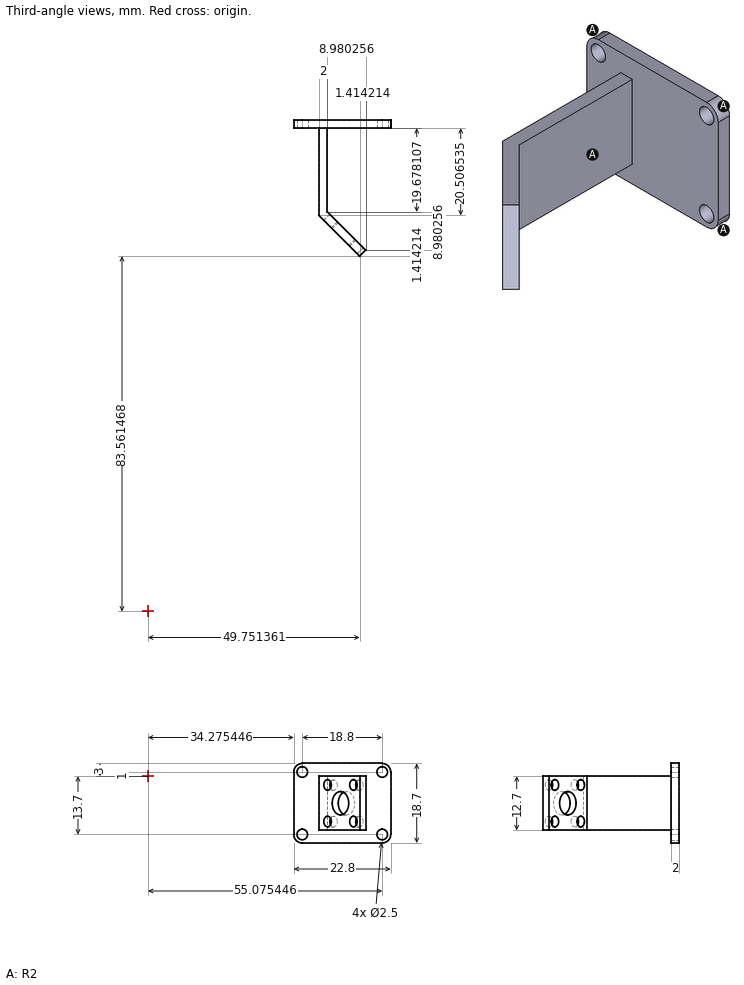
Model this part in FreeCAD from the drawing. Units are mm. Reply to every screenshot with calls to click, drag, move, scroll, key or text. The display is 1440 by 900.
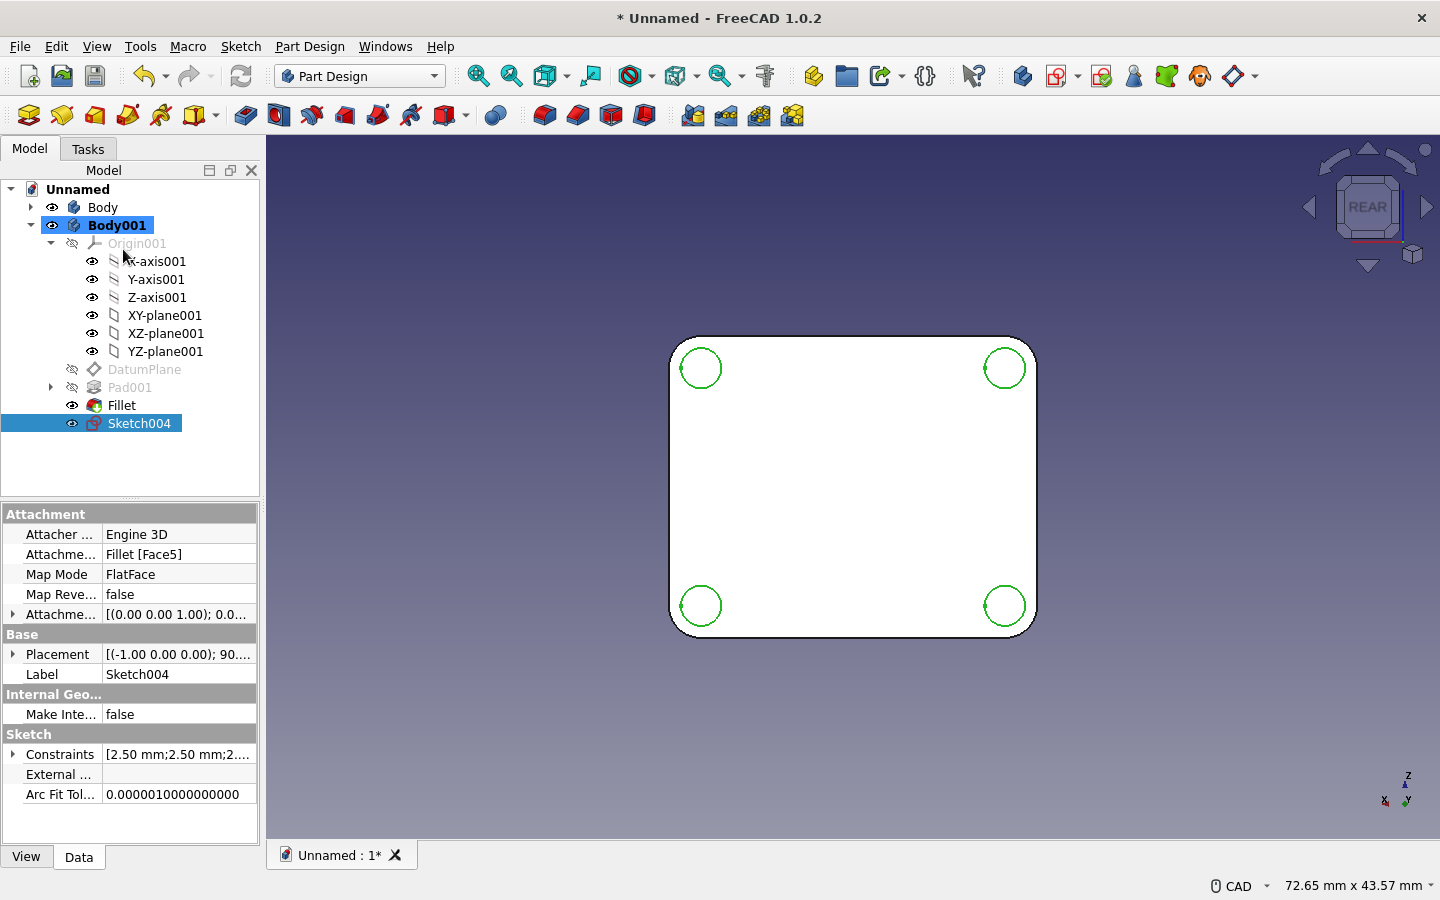
click(246, 116)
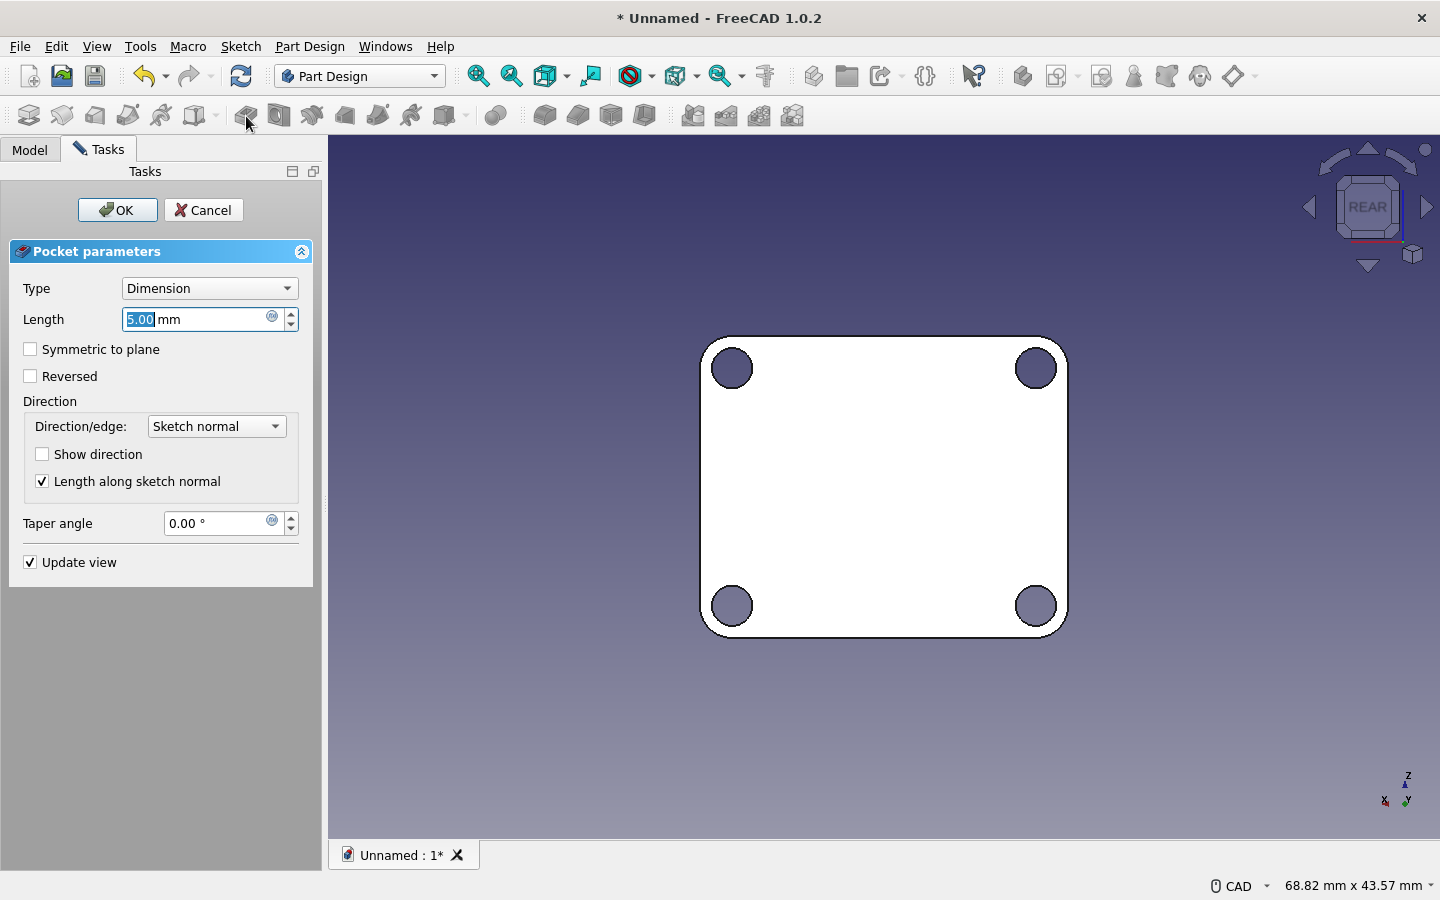
text(2)
key(Tab)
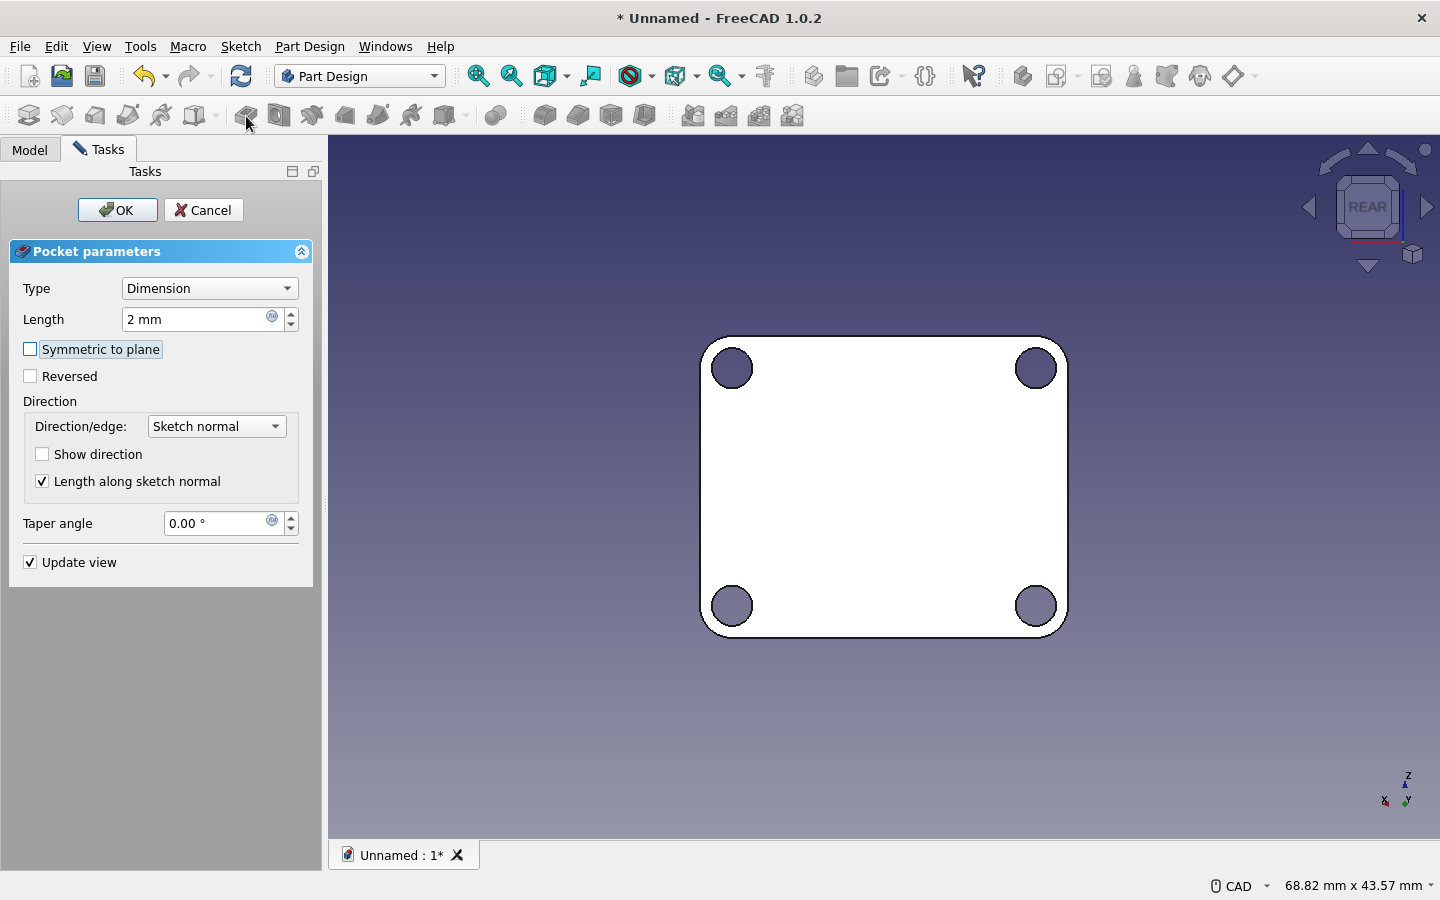
click(118, 210)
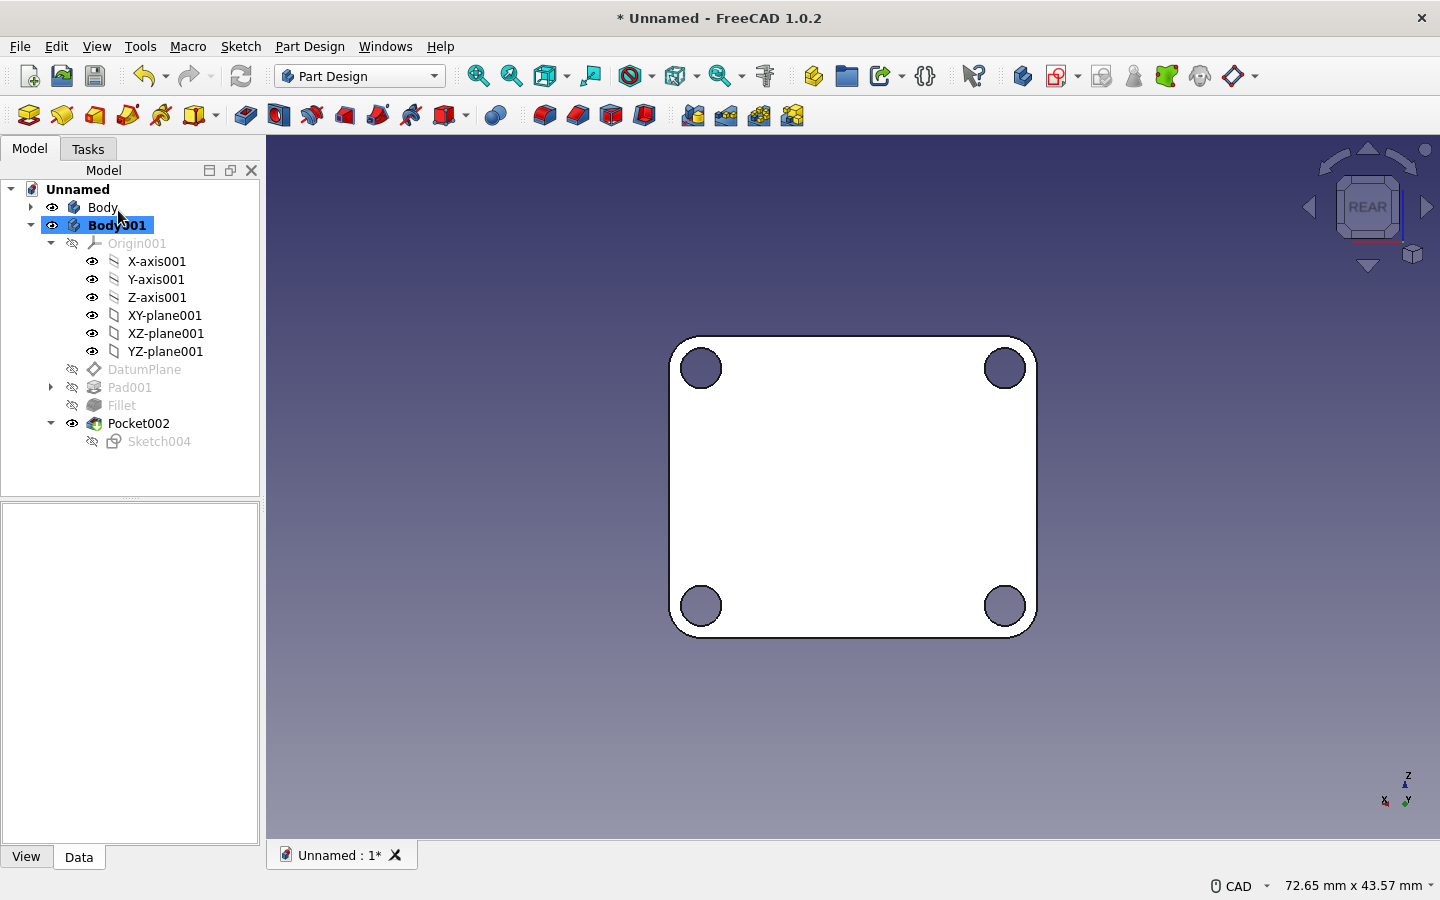
key(0)